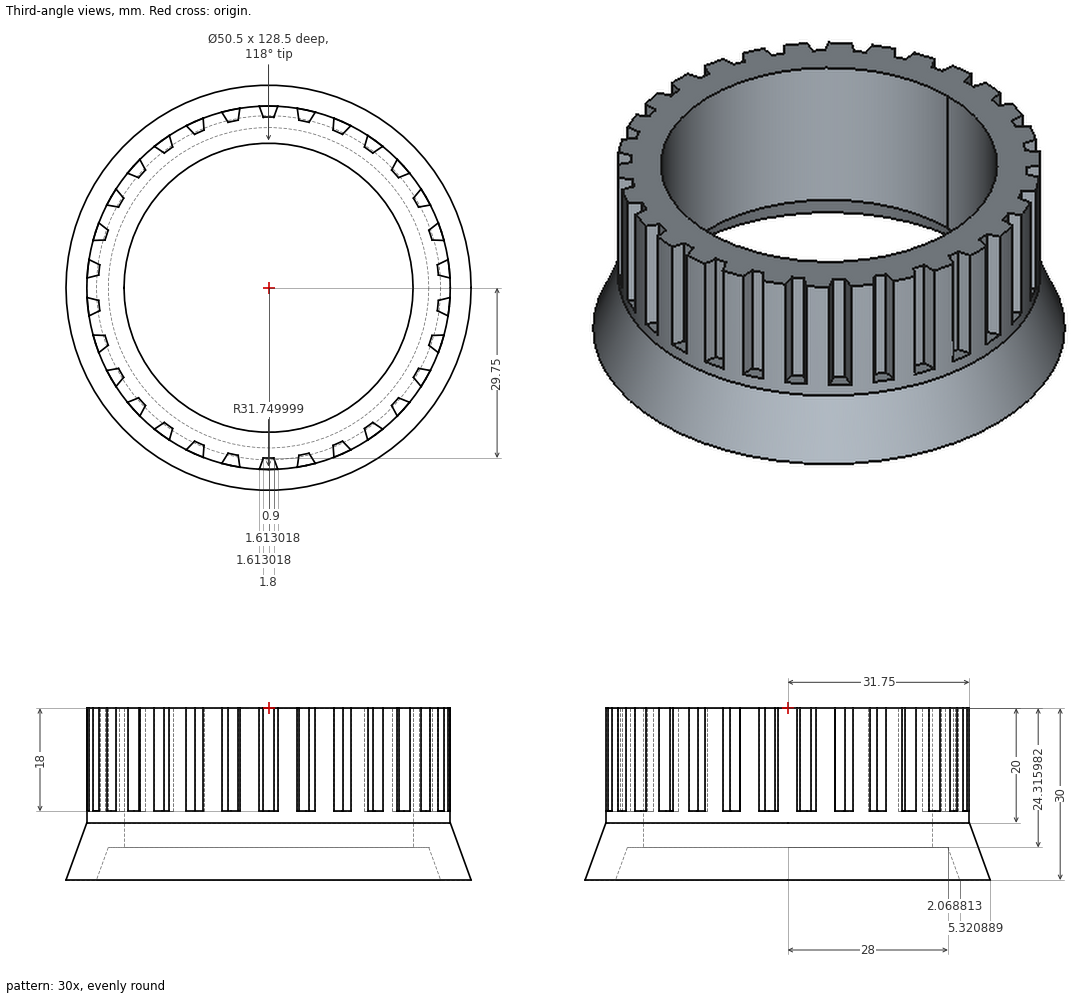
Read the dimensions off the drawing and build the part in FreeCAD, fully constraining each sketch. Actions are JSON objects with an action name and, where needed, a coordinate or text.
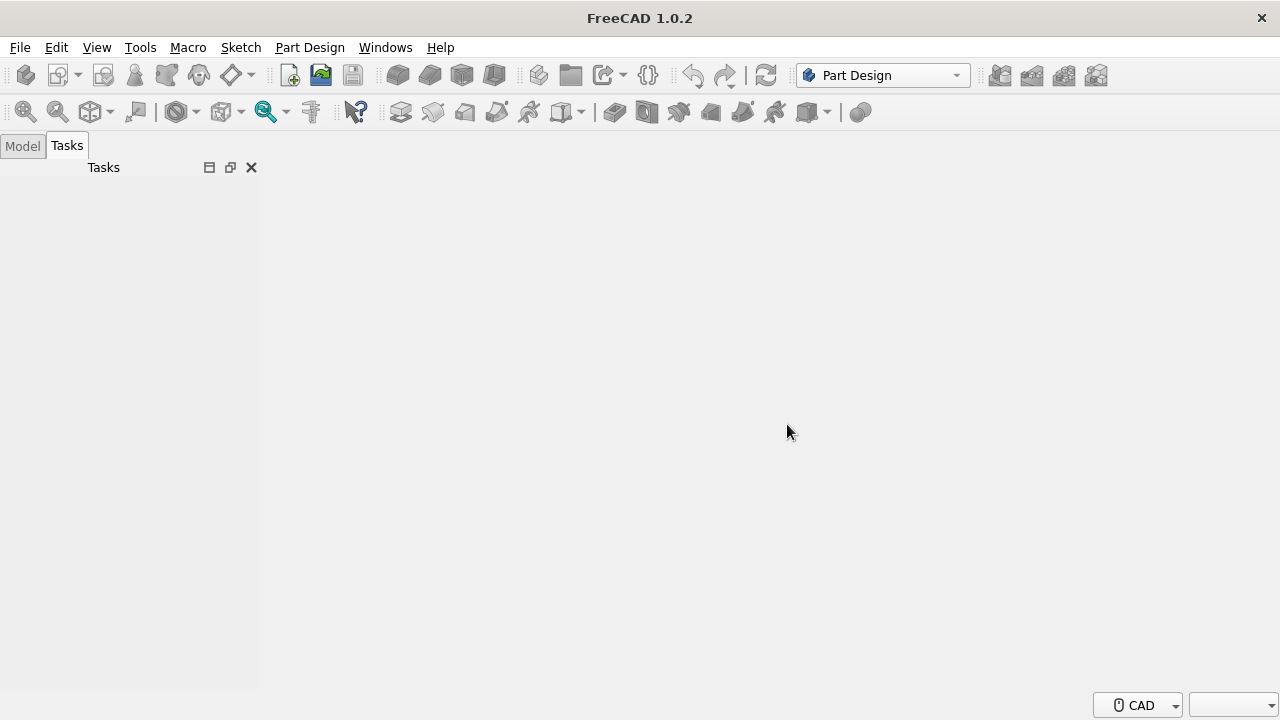
{"action": "left_click", "coordinate": [290, 76]}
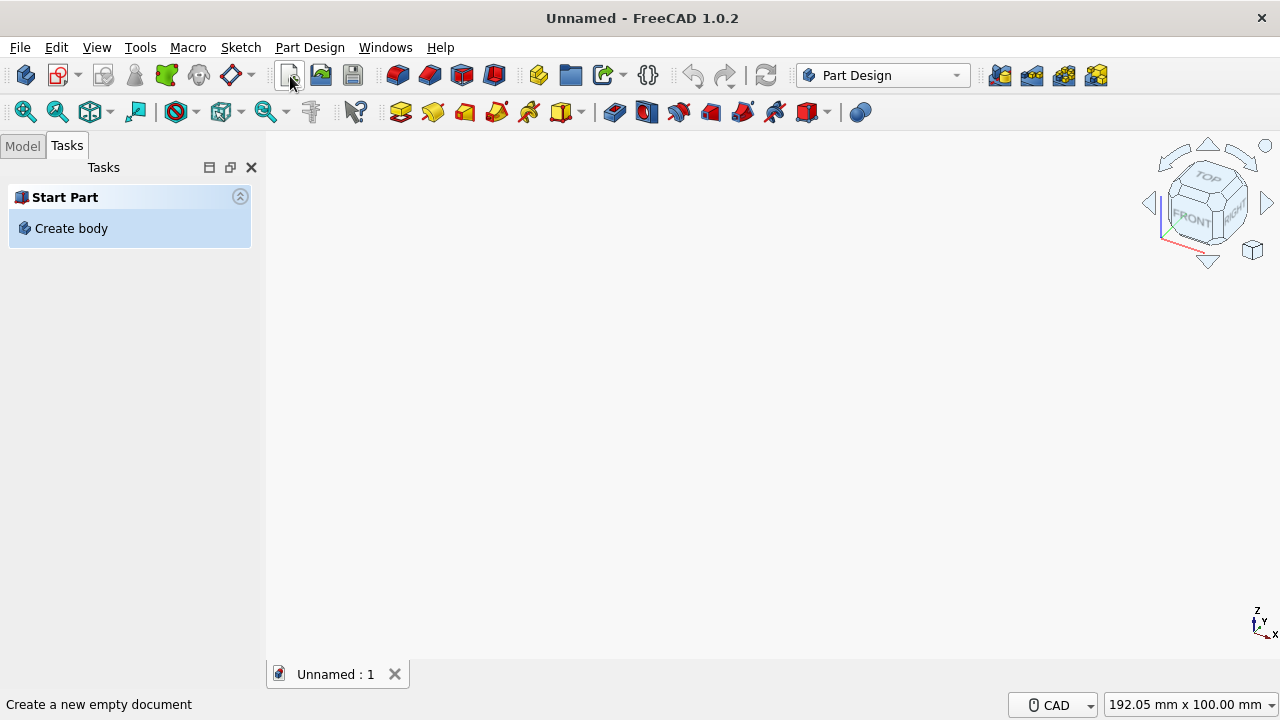
{"action": "left_click", "coordinate": [58, 76]}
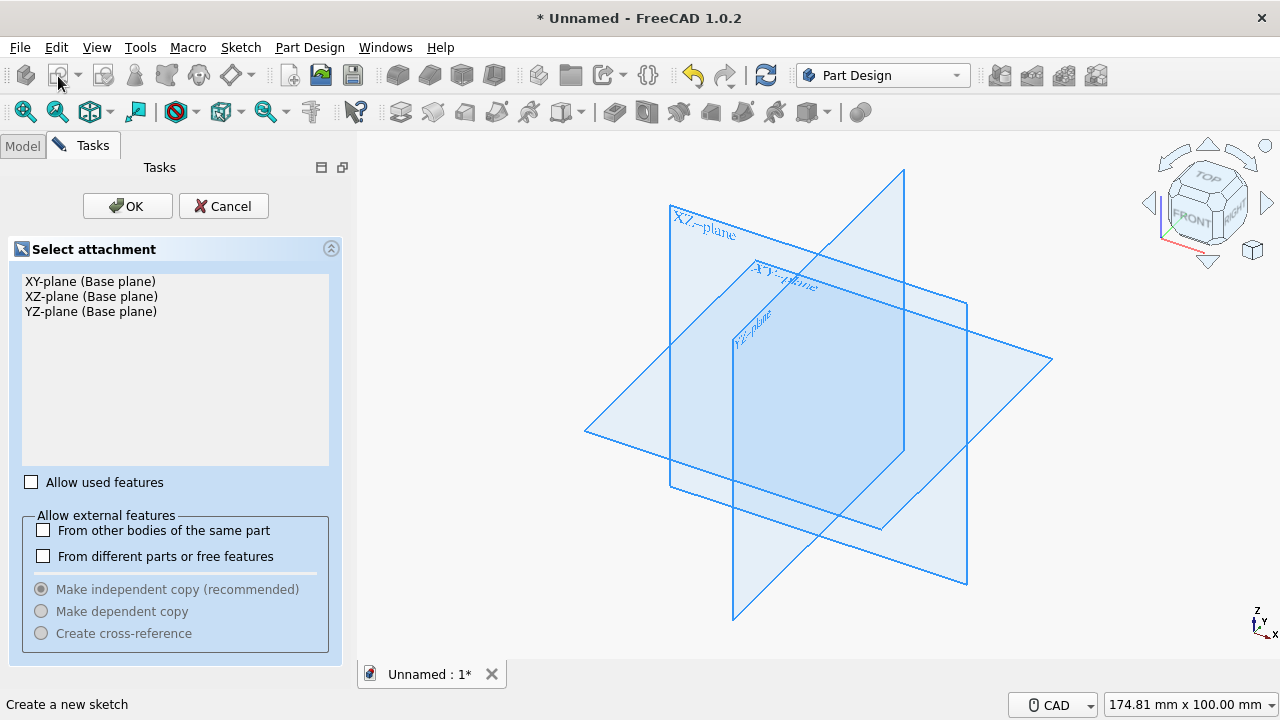
{"action": "left_click", "coordinate": [82, 312]}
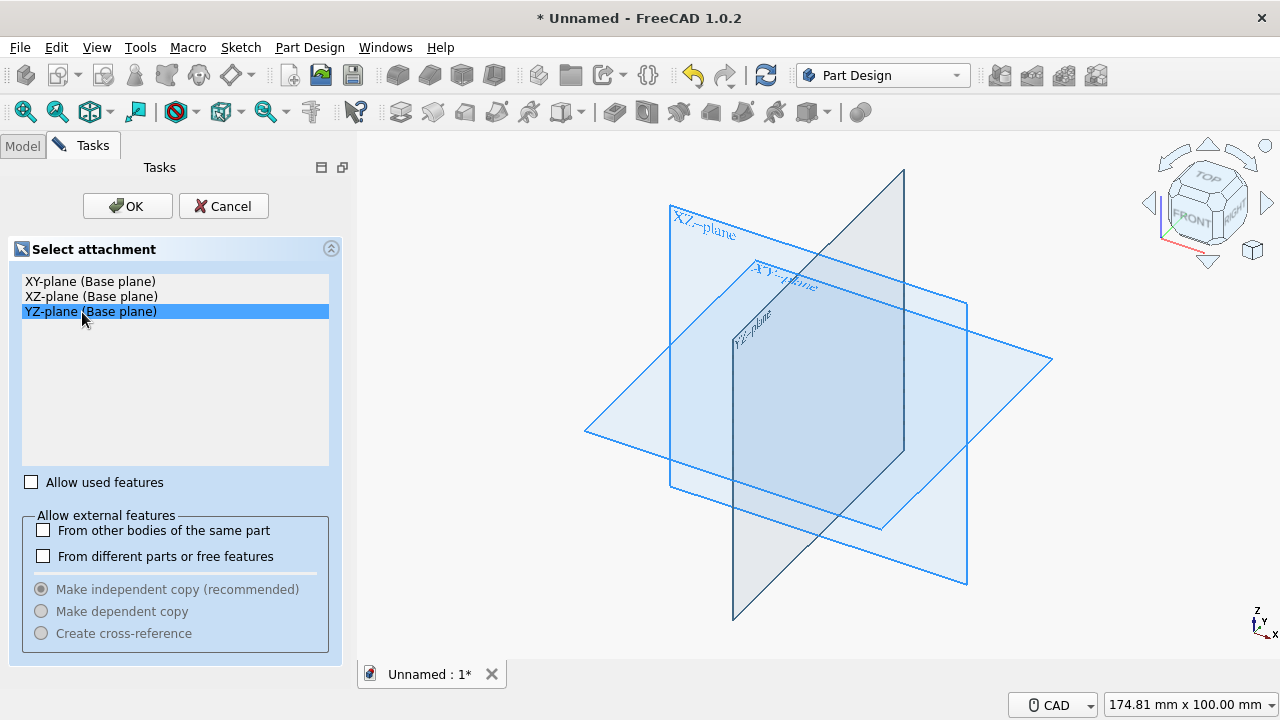
{"action": "left_click", "coordinate": [128, 206]}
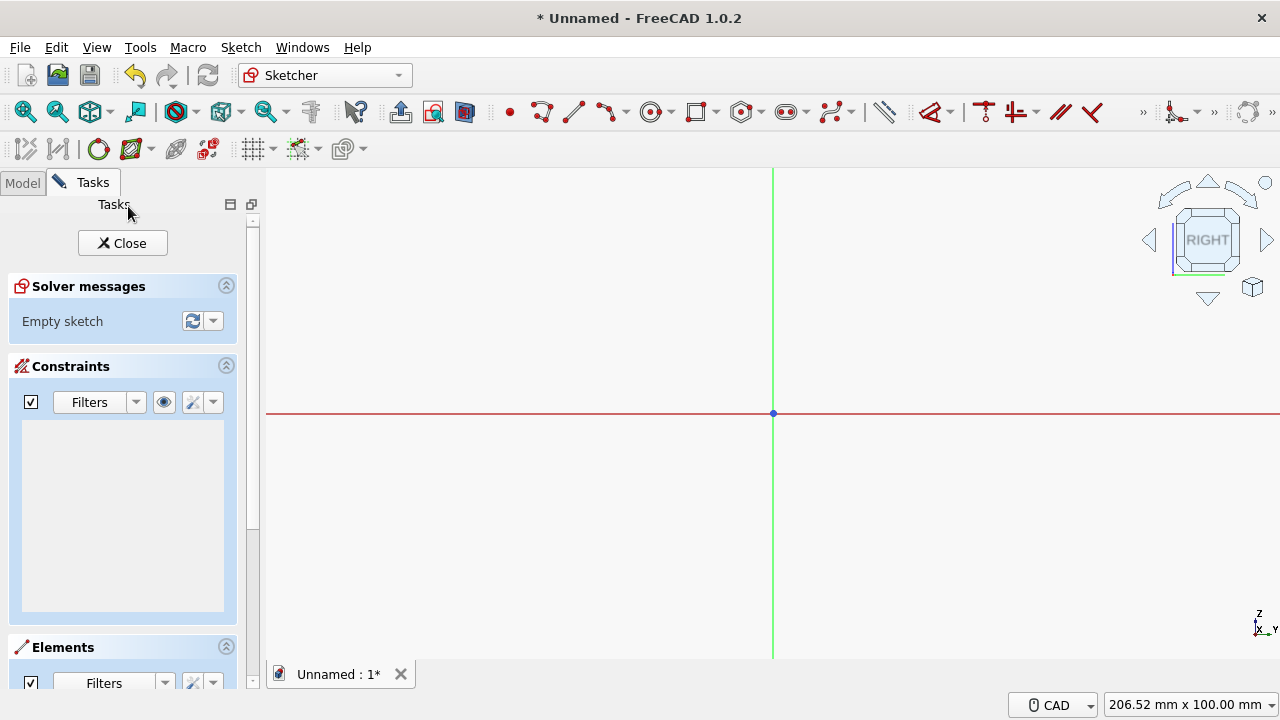
{"action": "scroll", "coordinate": [987, 547], "scroll_direction": "up", "scroll_amount": 4}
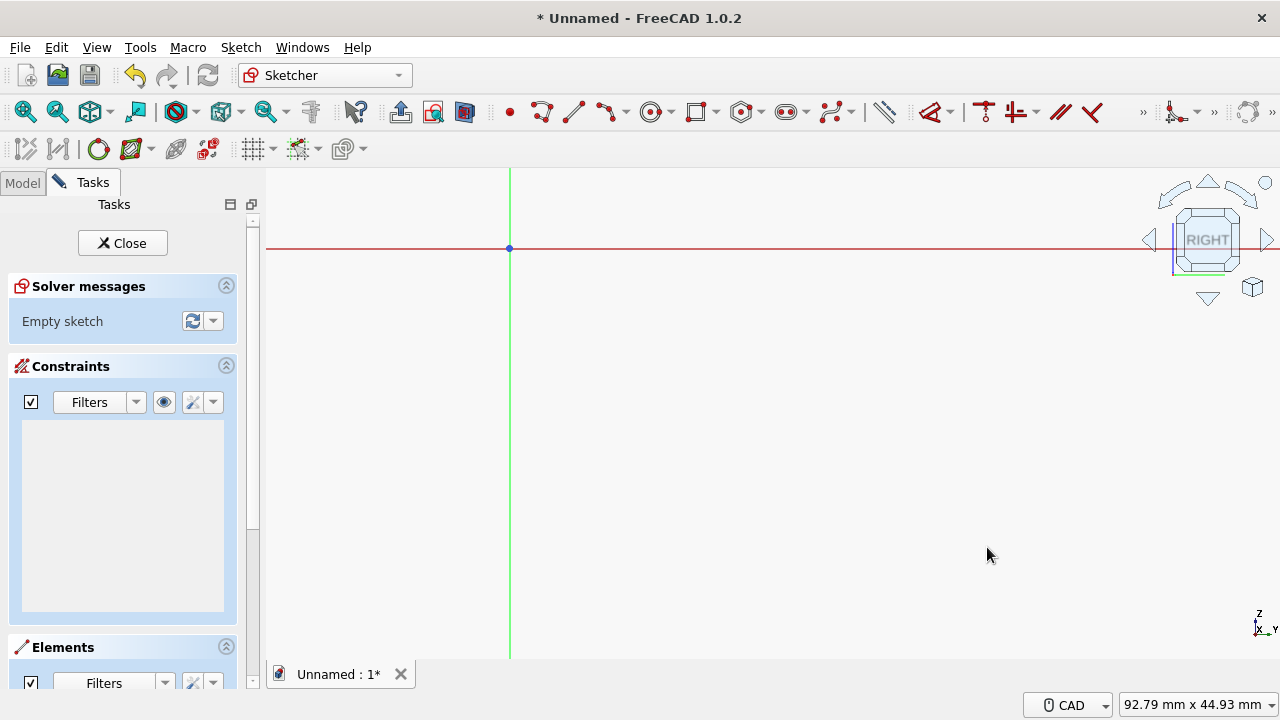
{"action": "left_click", "coordinate": [542, 112]}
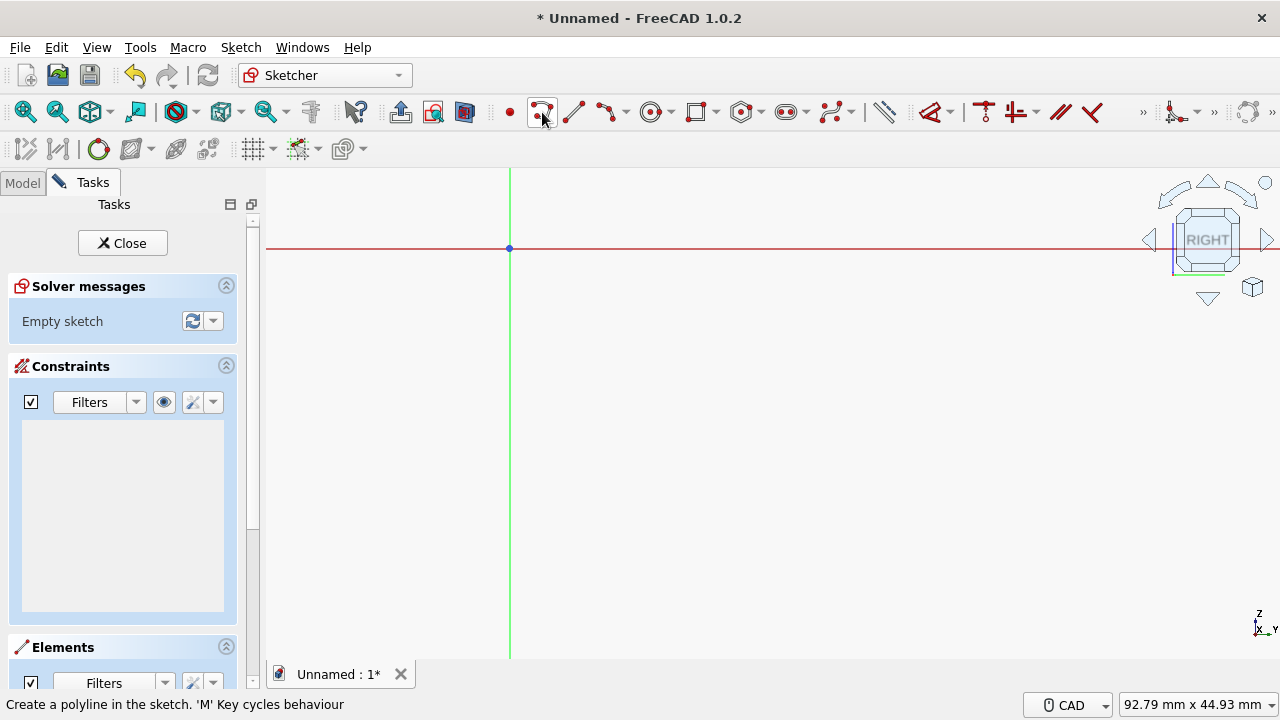
{"action": "left_click", "coordinate": [510, 249]}
{"action": "left_click", "coordinate": [519, 515]}
{"action": "left_click", "coordinate": [816, 515]}
{"action": "left_click", "coordinate": [838, 577]}
{"action": "left_click", "coordinate": [897, 577]}
{"action": "left_click", "coordinate": [857, 467]}
{"action": "left_click", "coordinate": [857, 258]}
{"action": "left_click", "coordinate": [510, 249]}
{"action": "key", "text": "Escape"}
{"action": "key", "text": "Escape"}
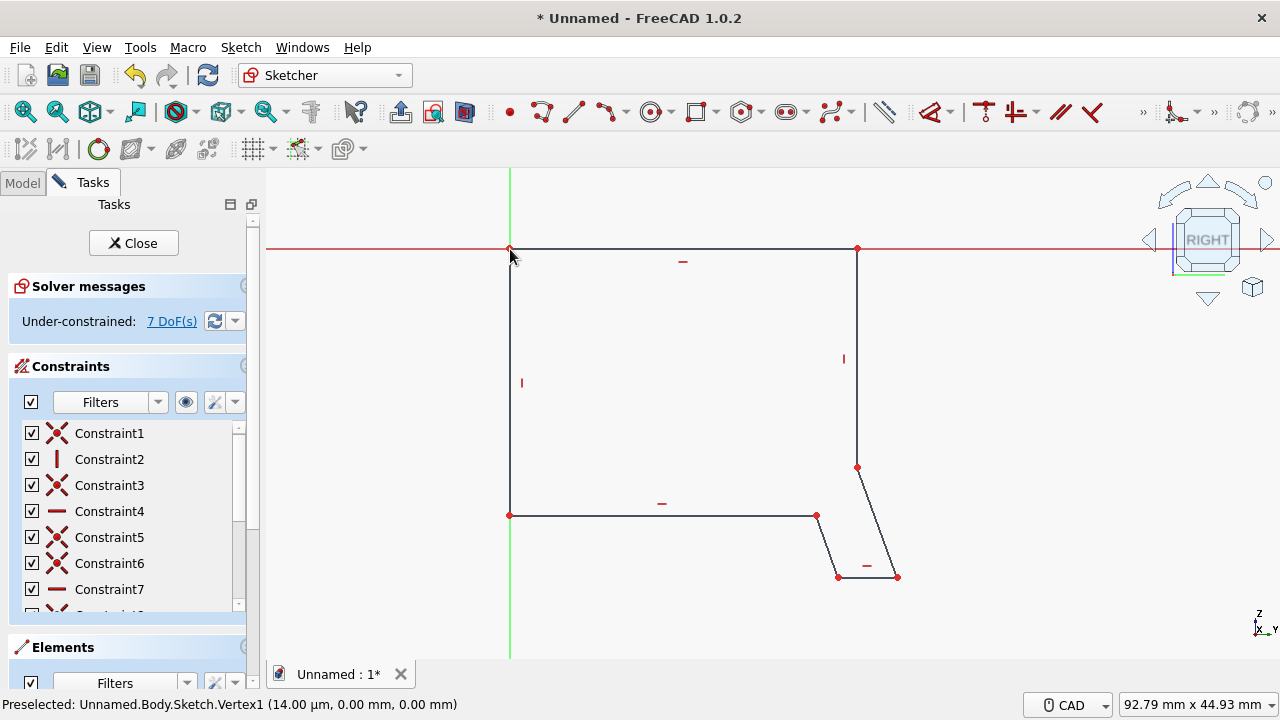
{"action": "left_click", "coordinate": [930, 112]}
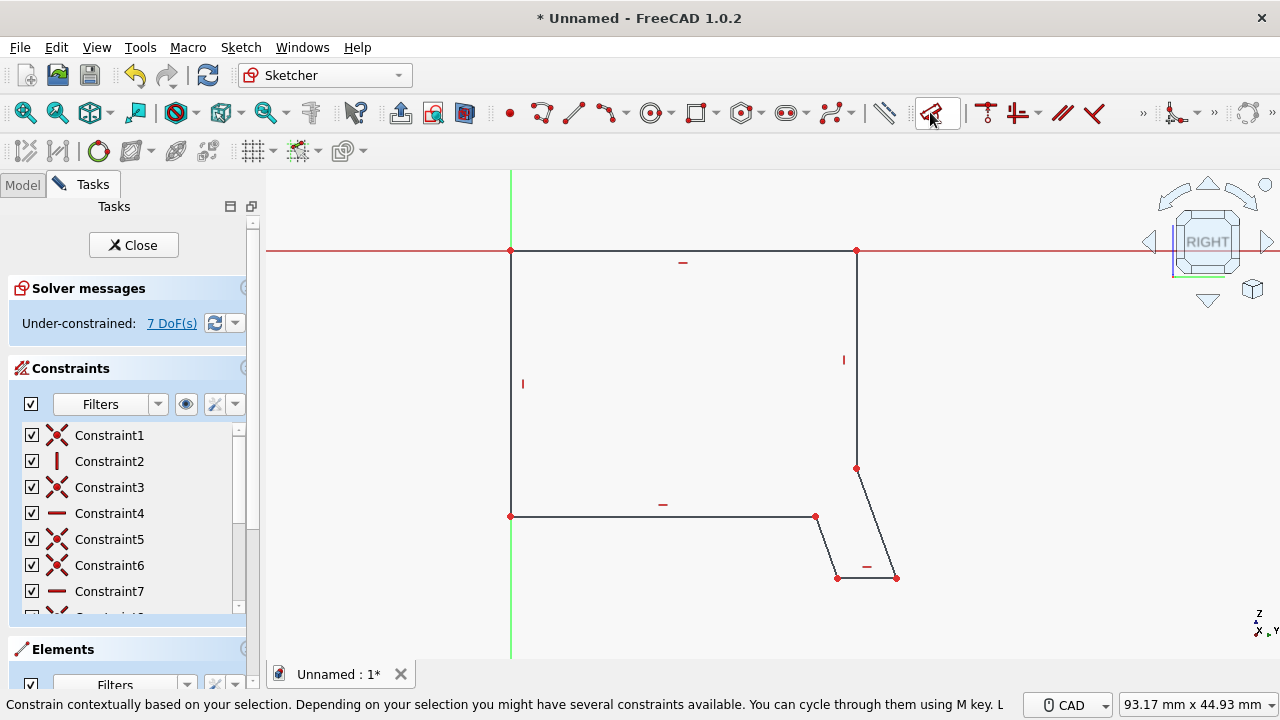
{"action": "left_click", "coordinate": [602, 517]}
{"action": "left_click", "coordinate": [663, 551]}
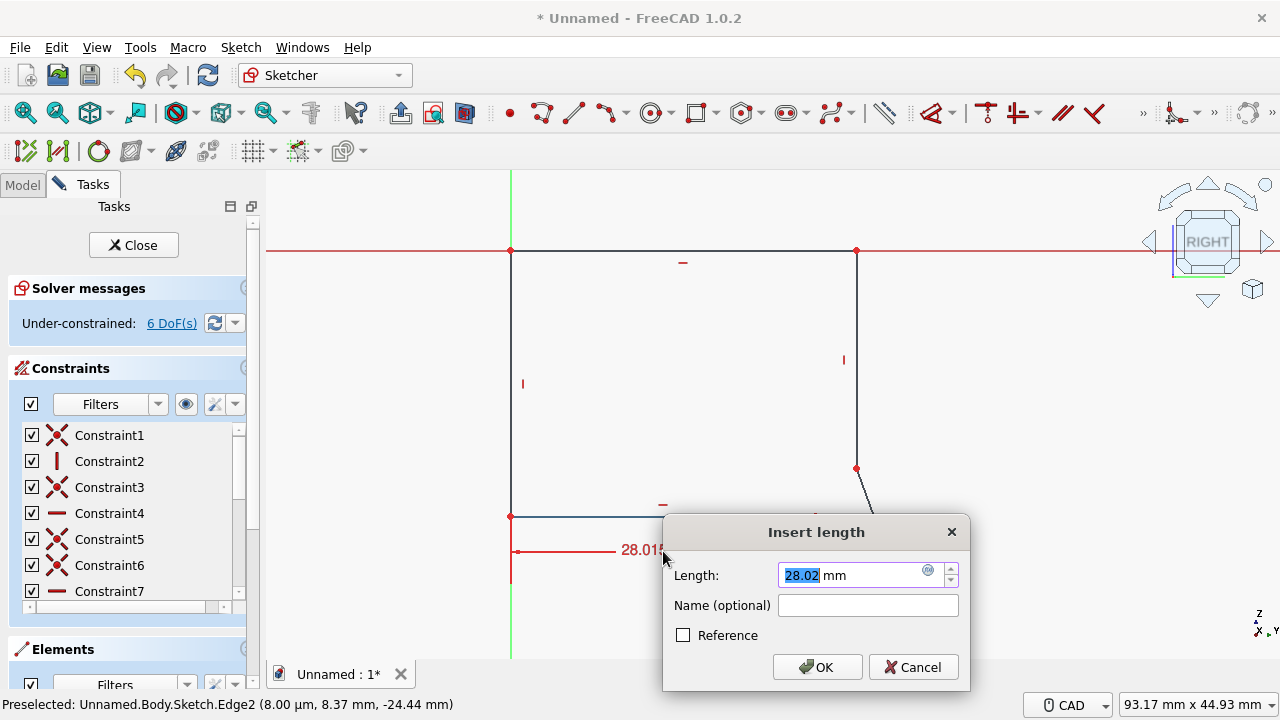
{"action": "type", "text": "28"}
{"action": "key", "text": "Return"}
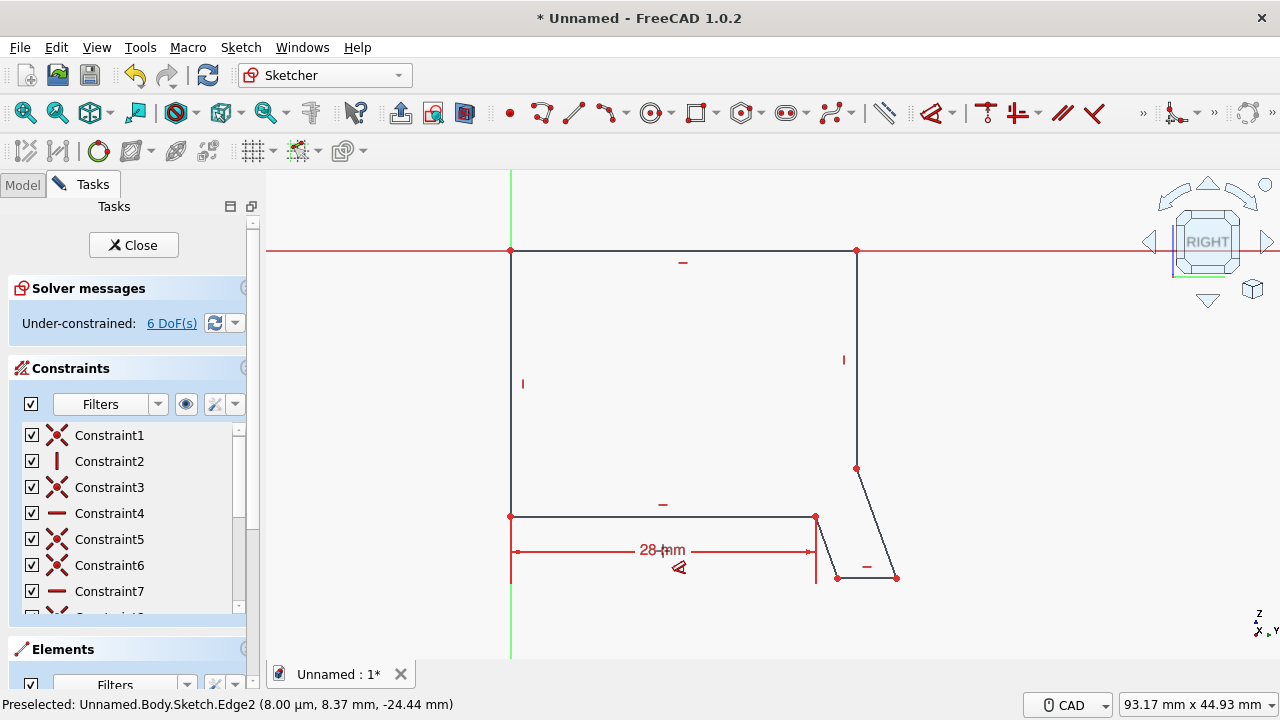
{"action": "left_click", "coordinate": [857, 403]}
{"action": "left_click", "coordinate": [891, 360]}